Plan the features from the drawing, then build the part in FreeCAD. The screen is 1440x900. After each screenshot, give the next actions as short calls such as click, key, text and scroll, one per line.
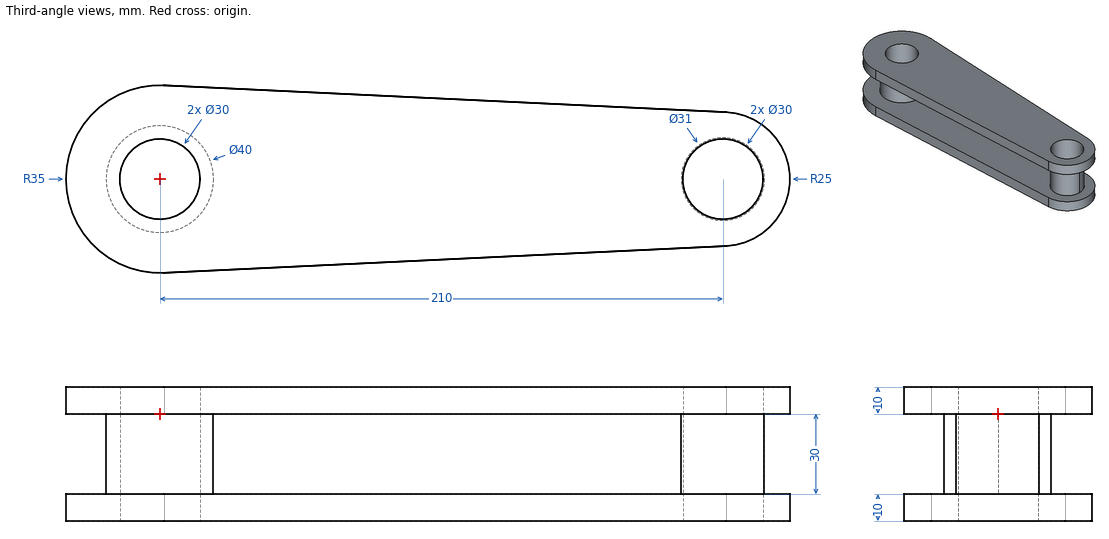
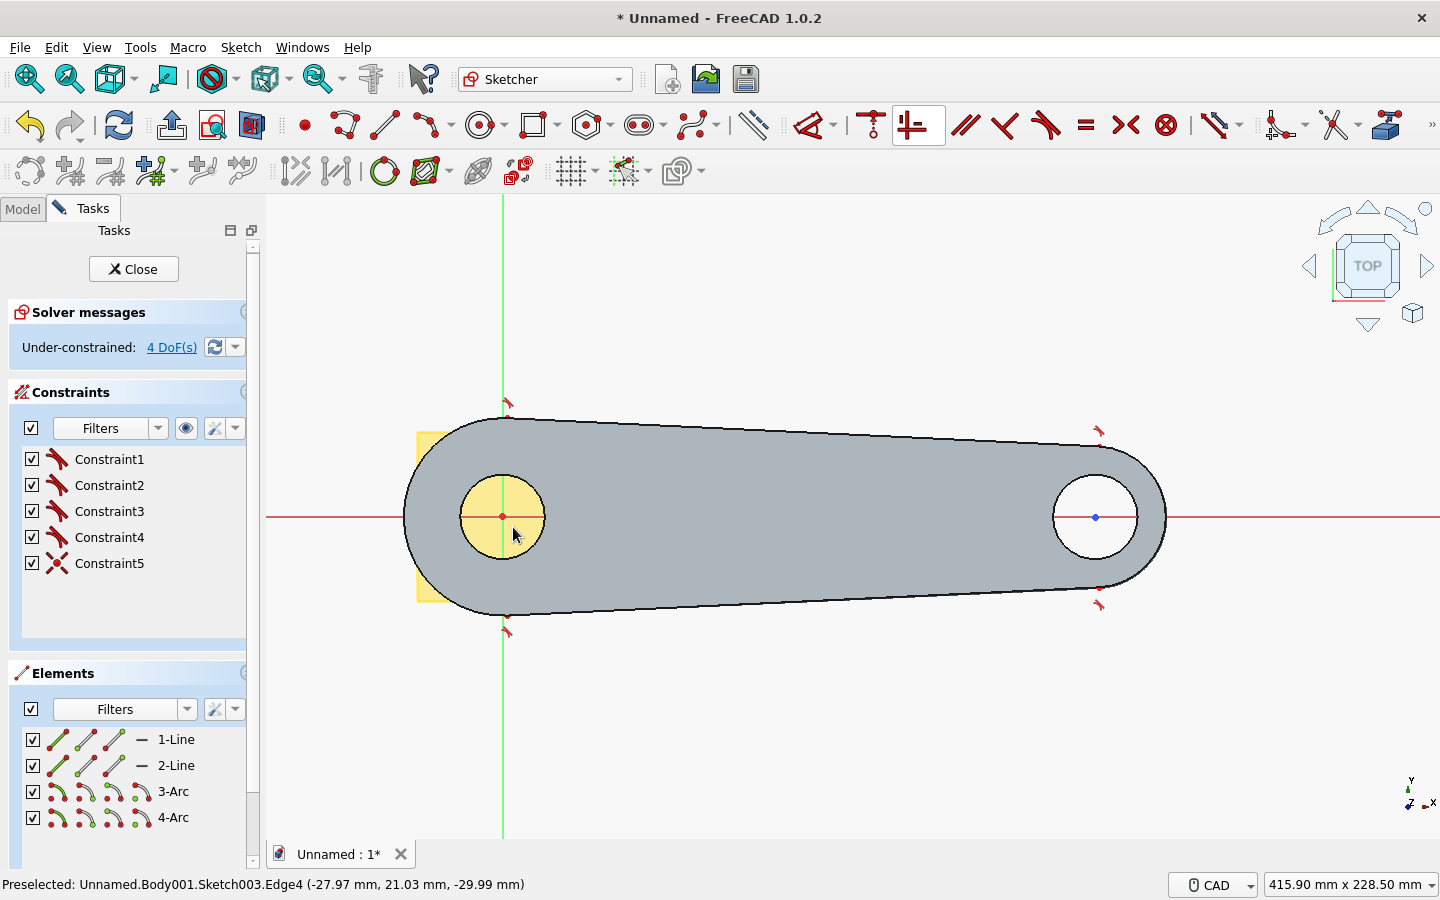
click(1096, 517)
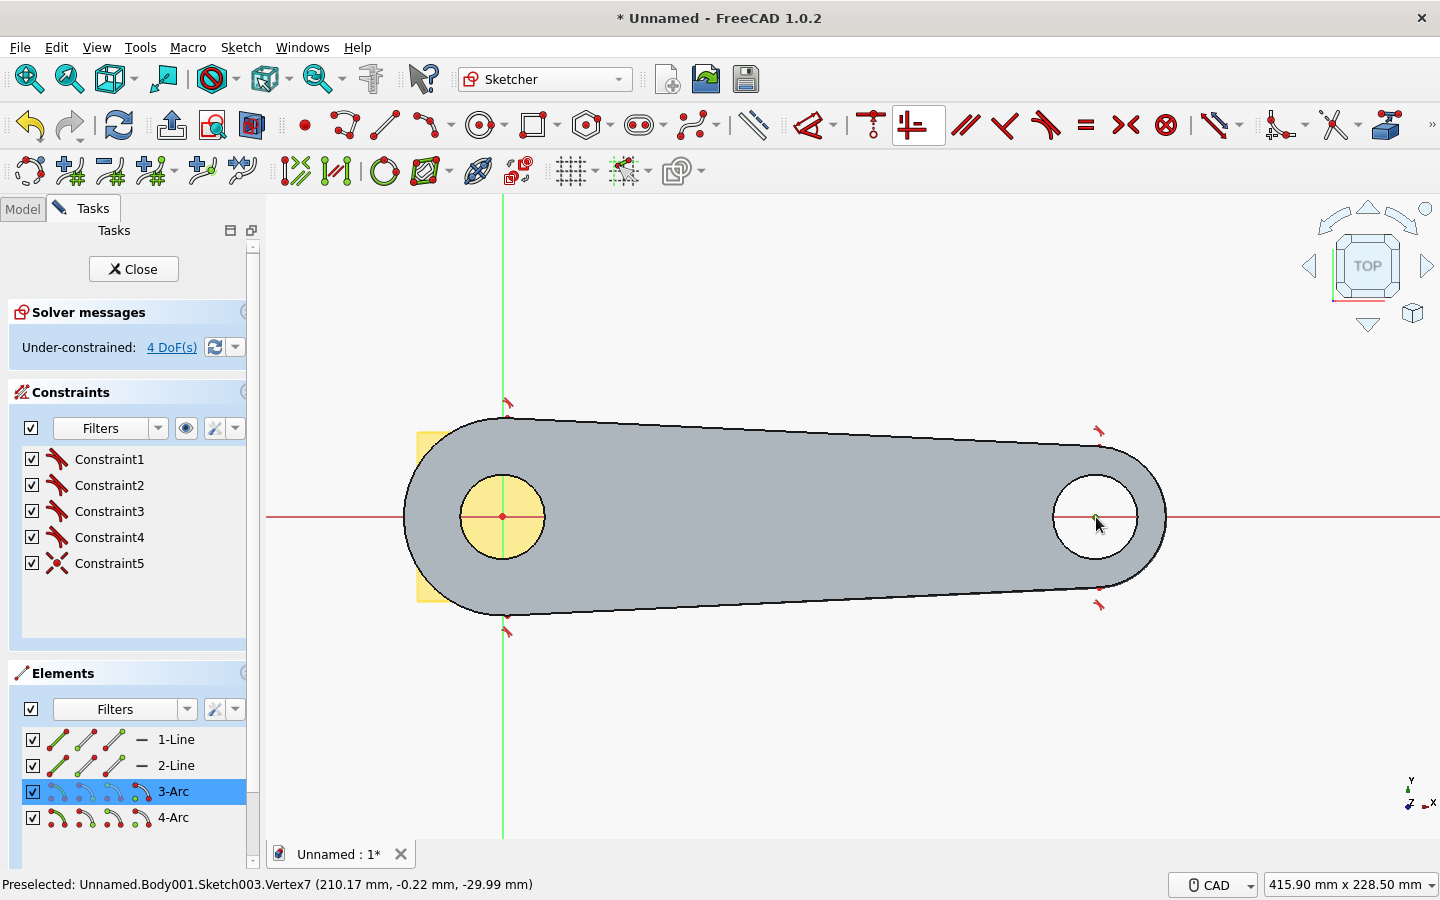
click(364, 517)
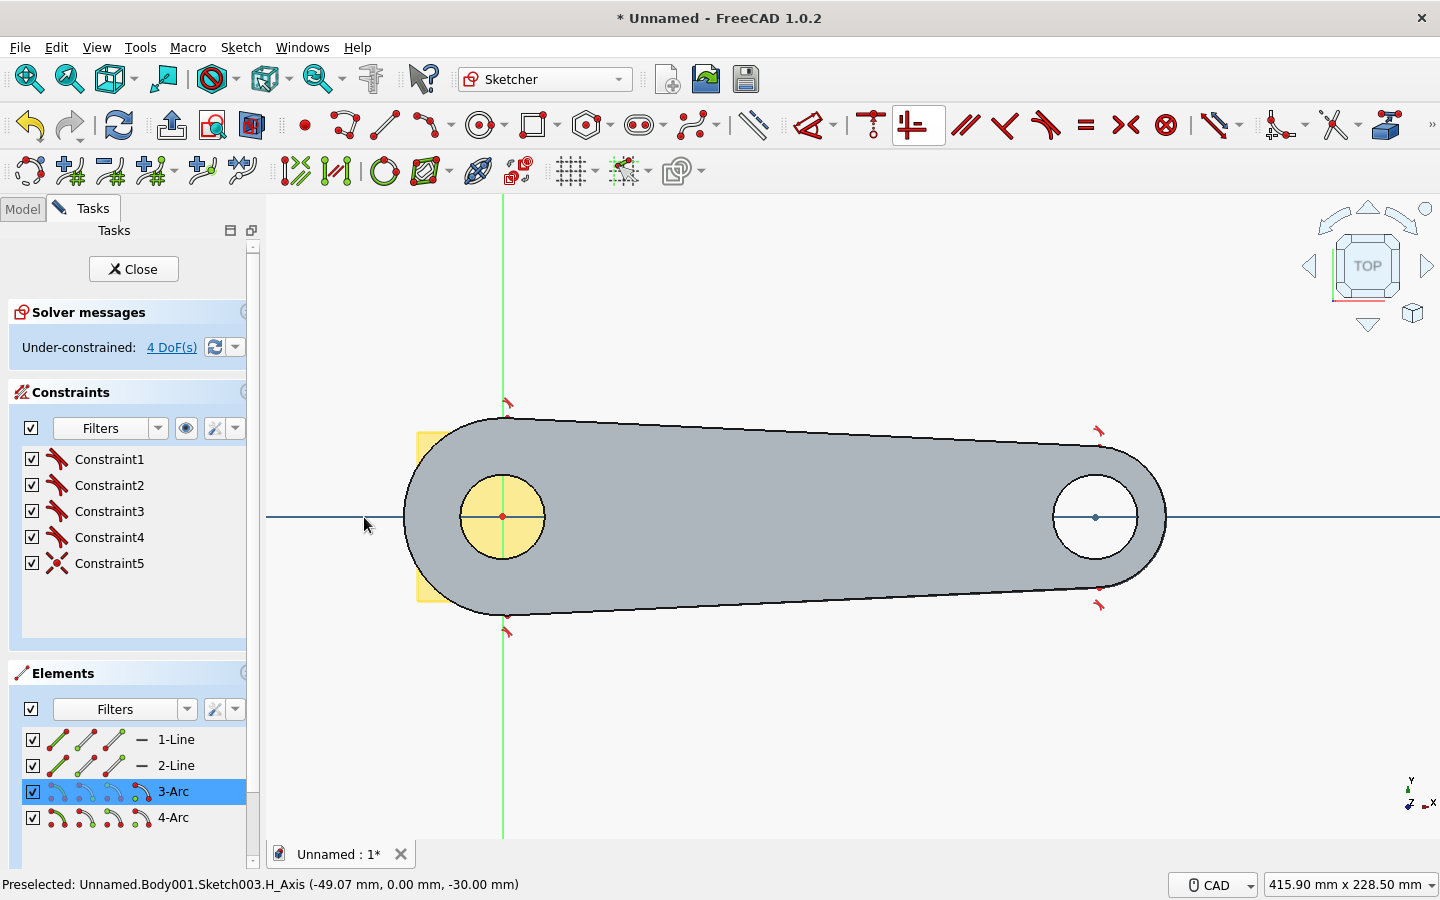
click(872, 126)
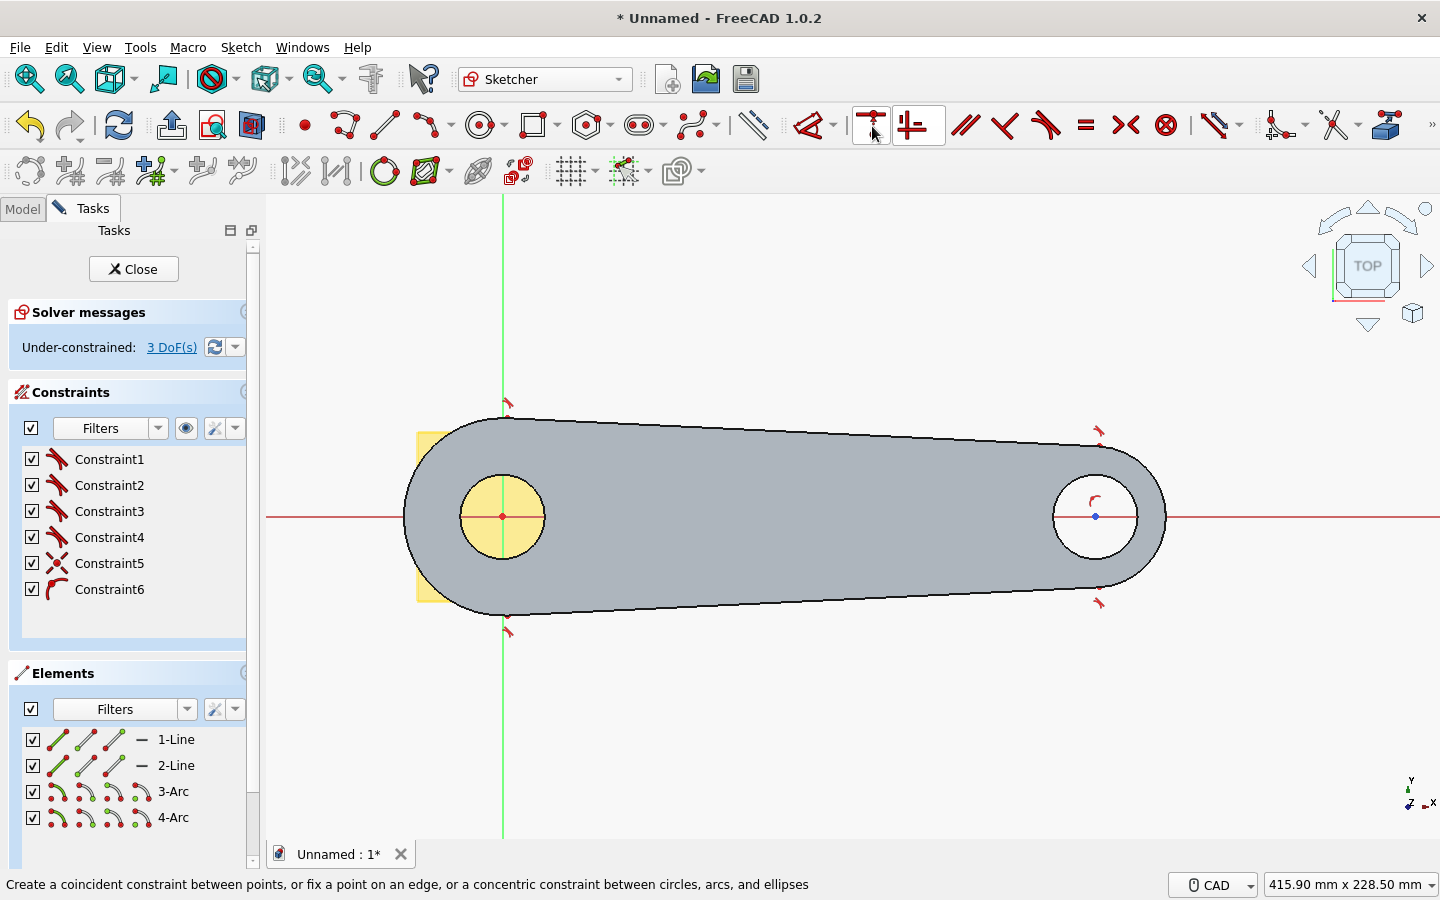
click(808, 126)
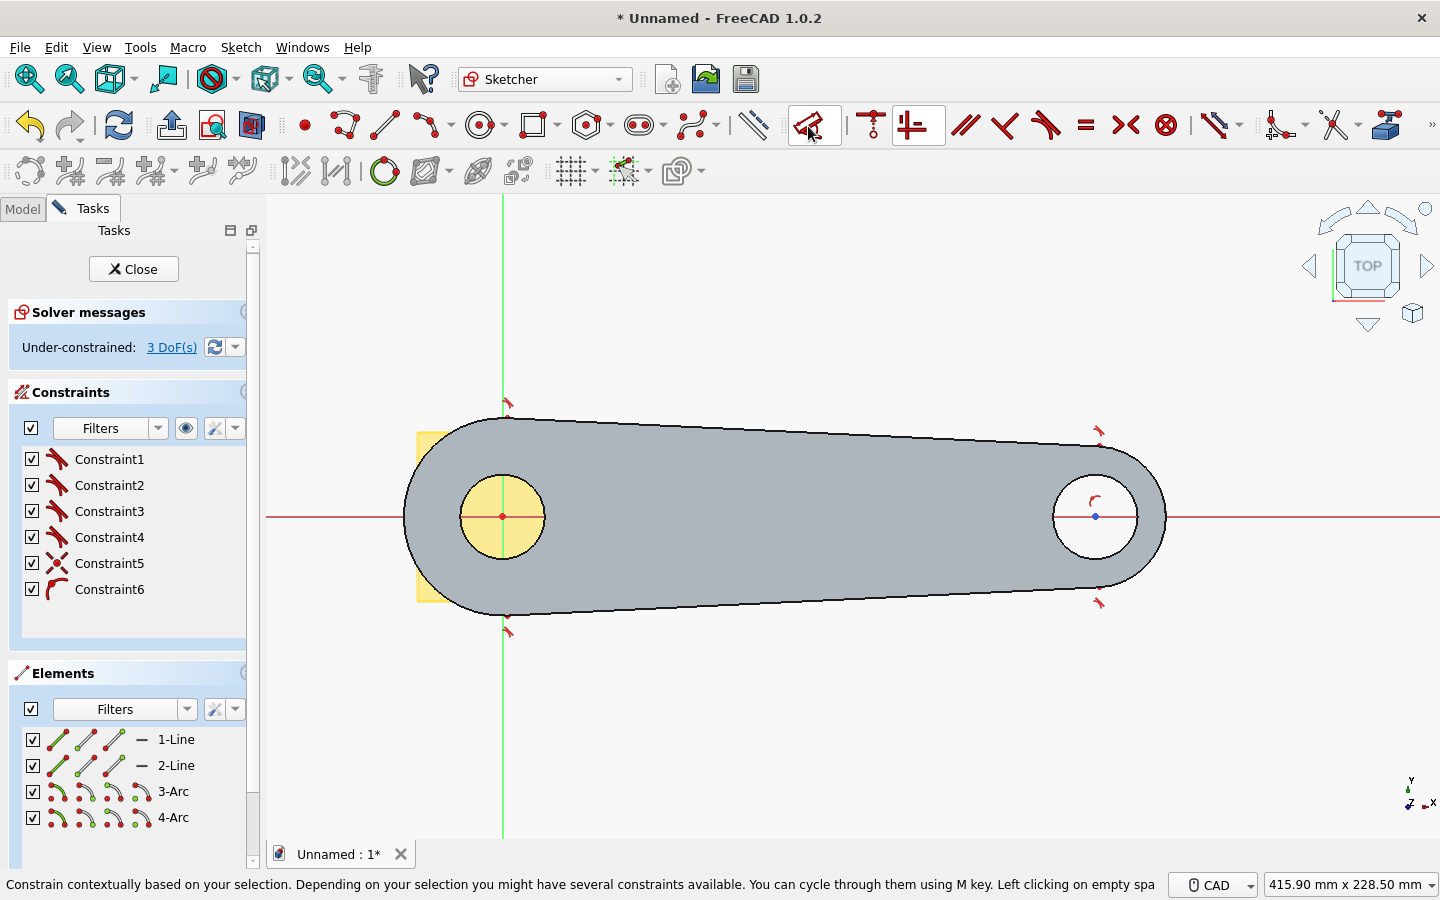
click(1153, 557)
click(1179, 575)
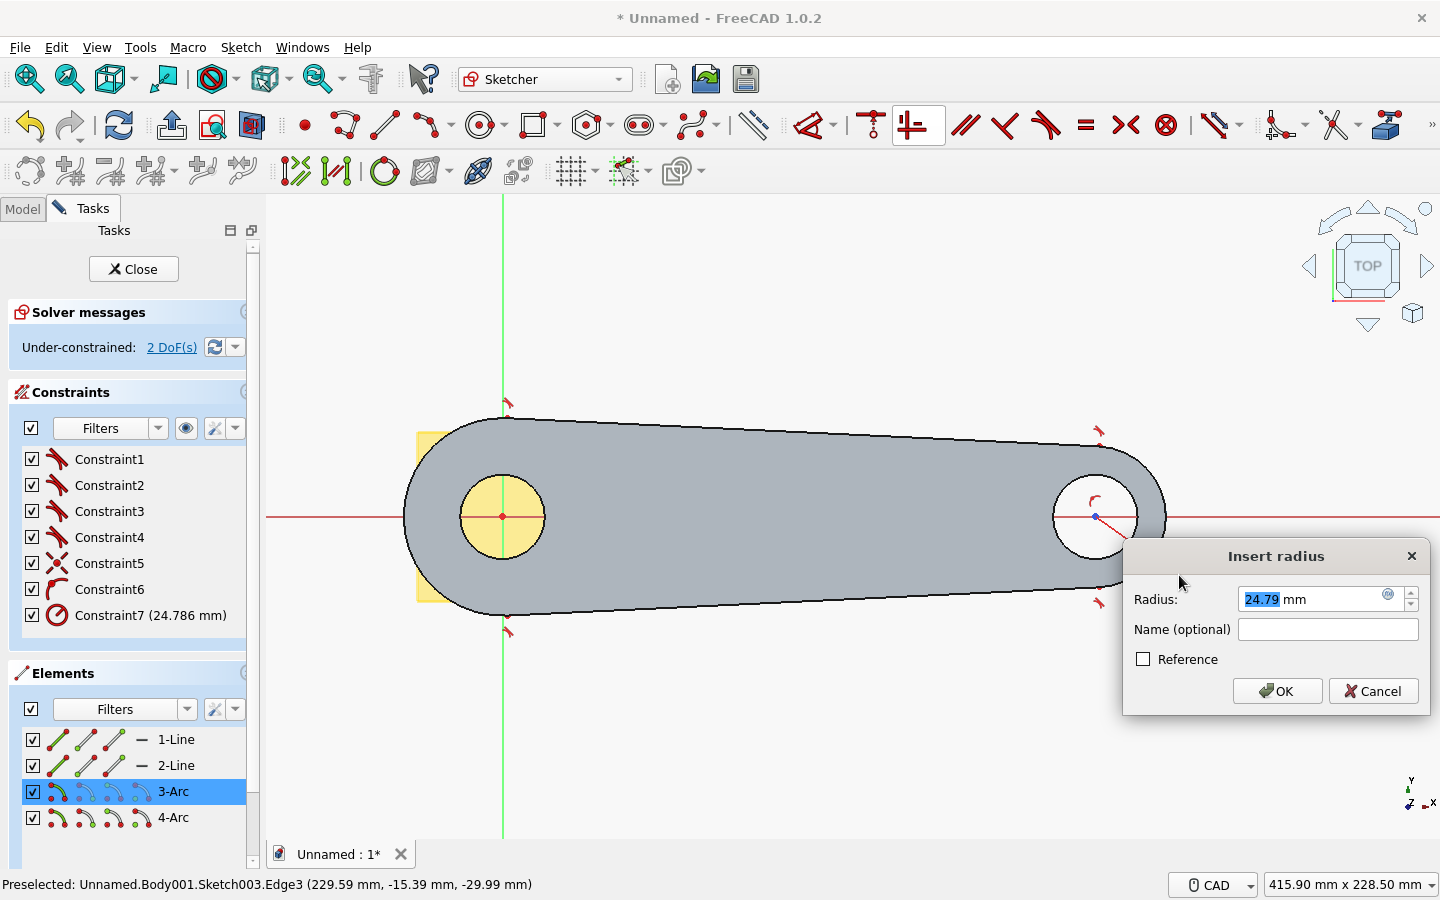
text(25)
key(Return)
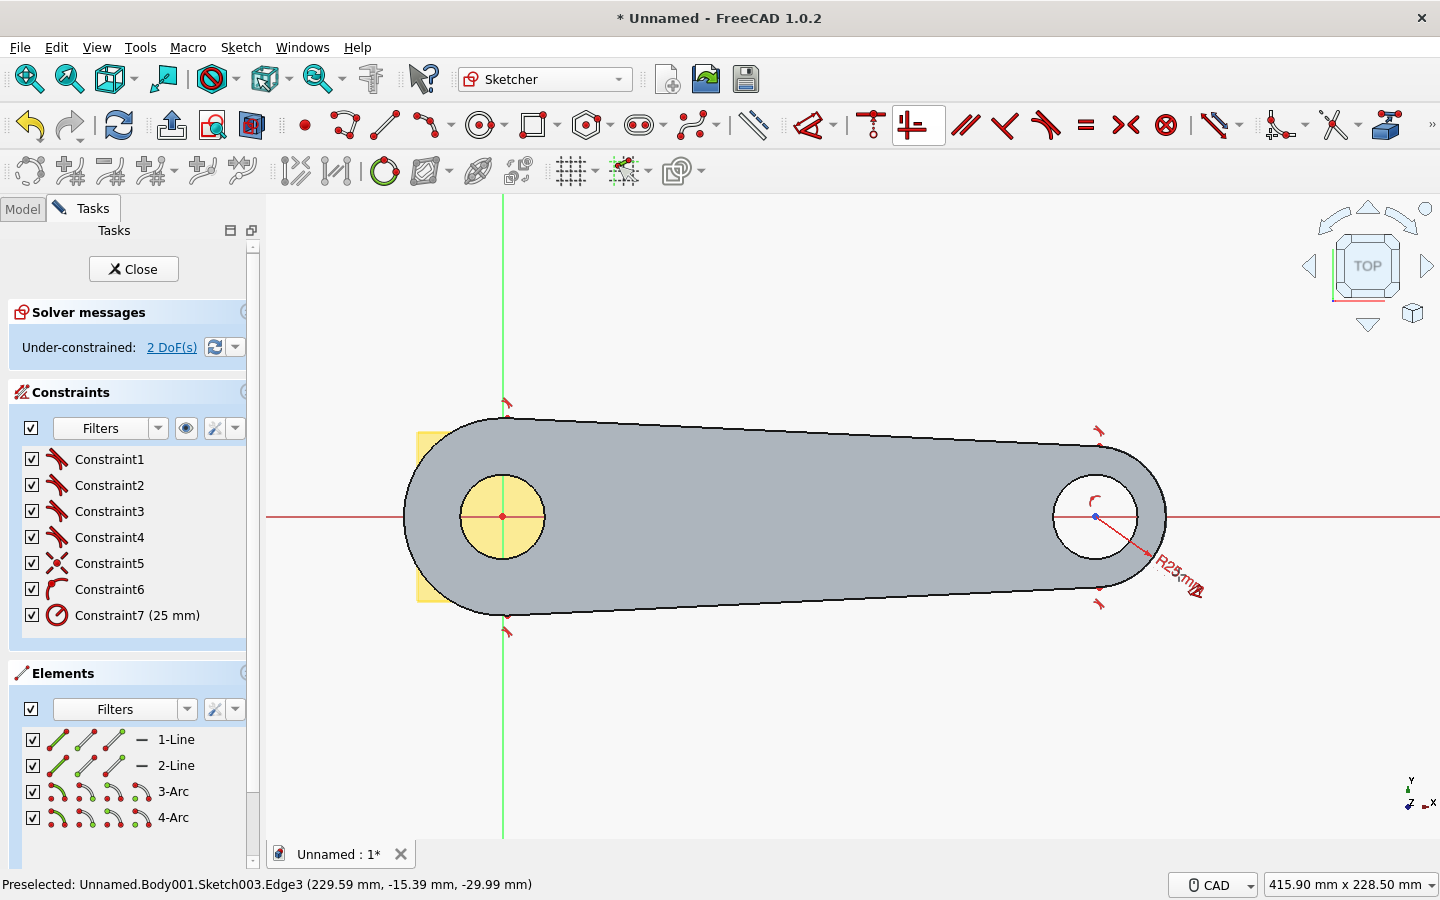
click(424, 457)
click(399, 438)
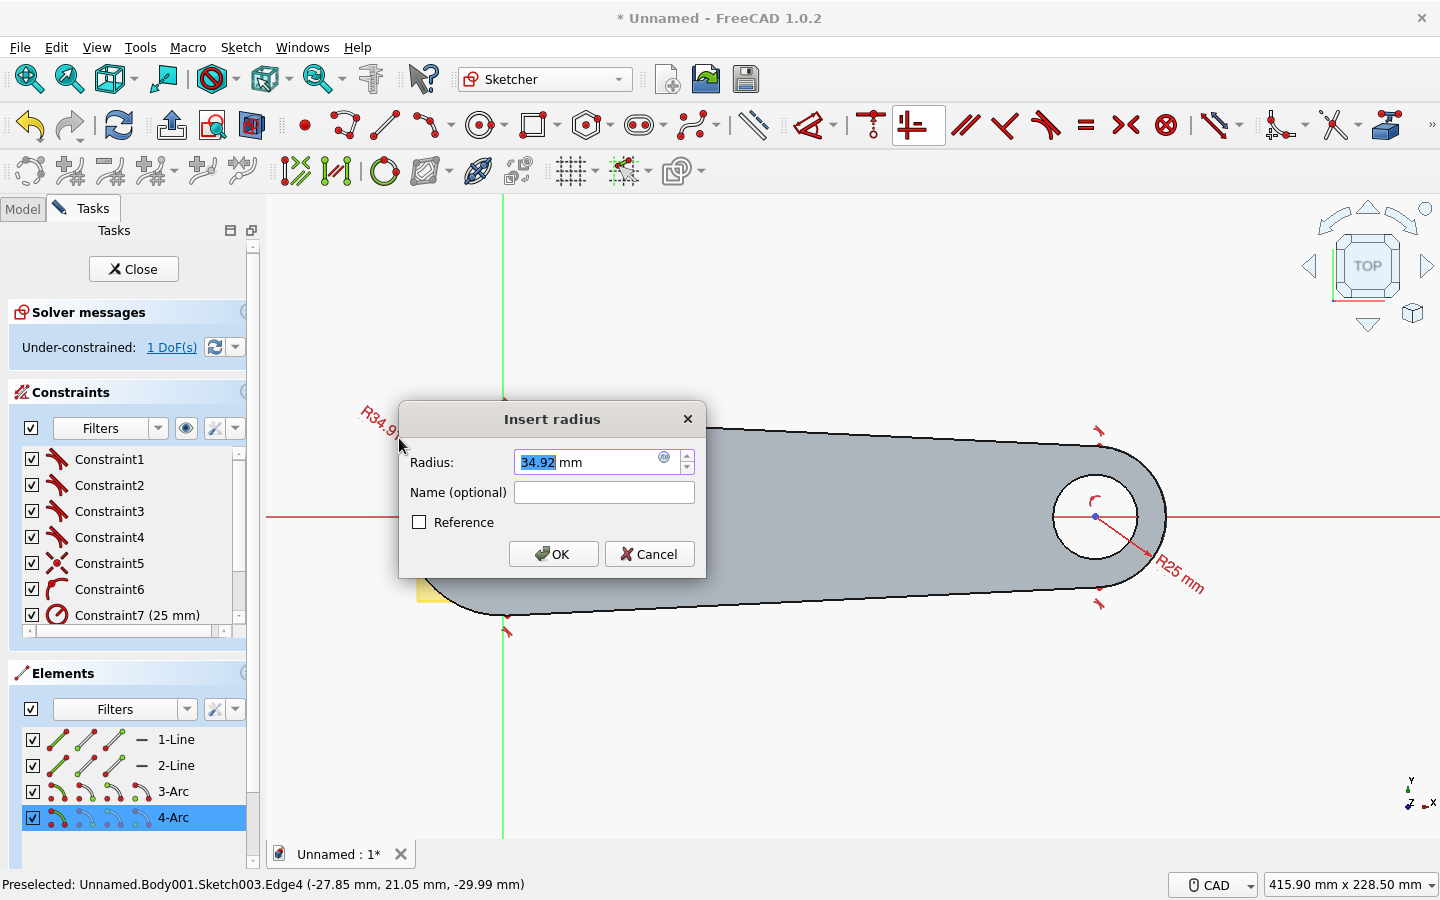
text(35)
key(Return)